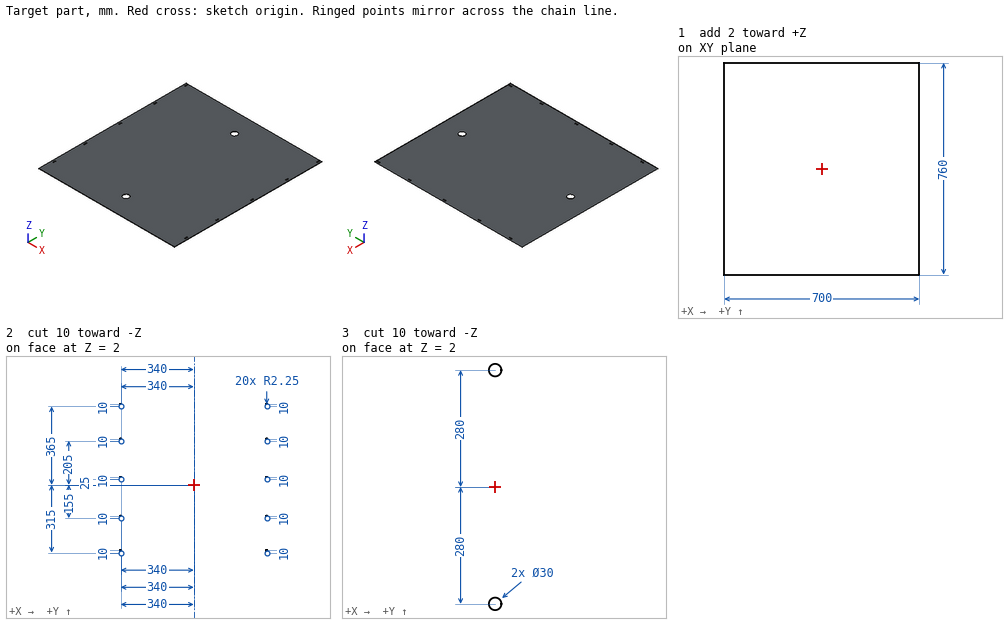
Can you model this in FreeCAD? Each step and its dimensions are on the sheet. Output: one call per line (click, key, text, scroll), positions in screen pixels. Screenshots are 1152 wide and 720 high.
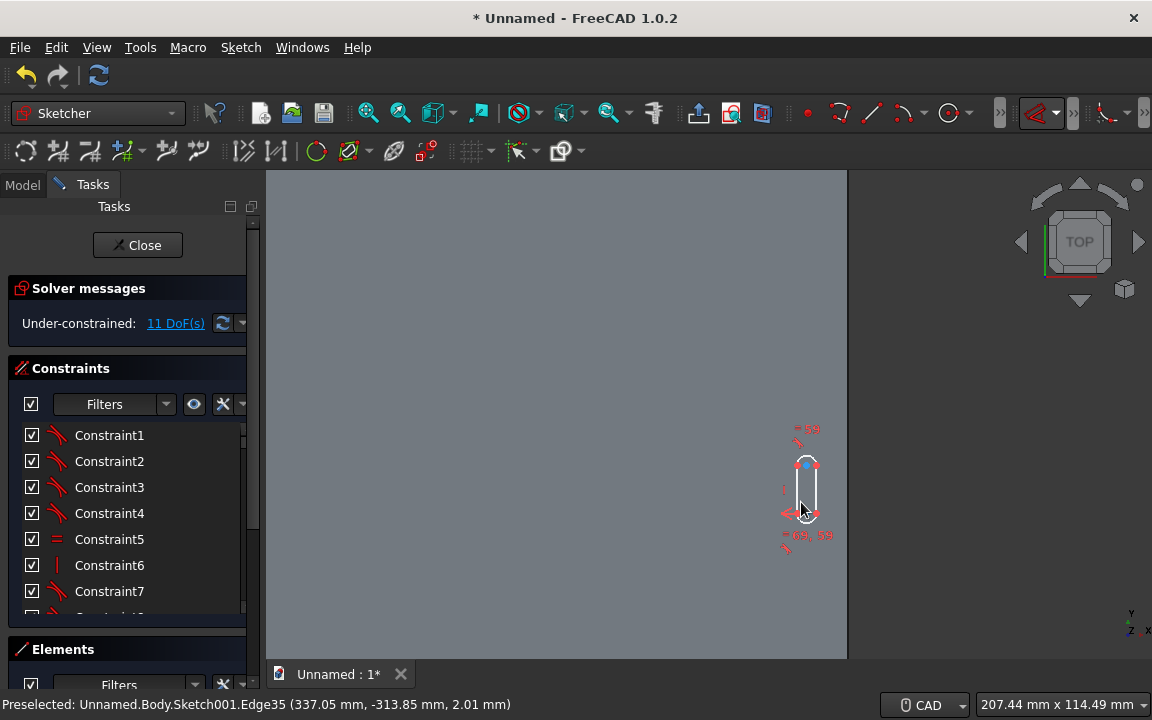
click(797, 499)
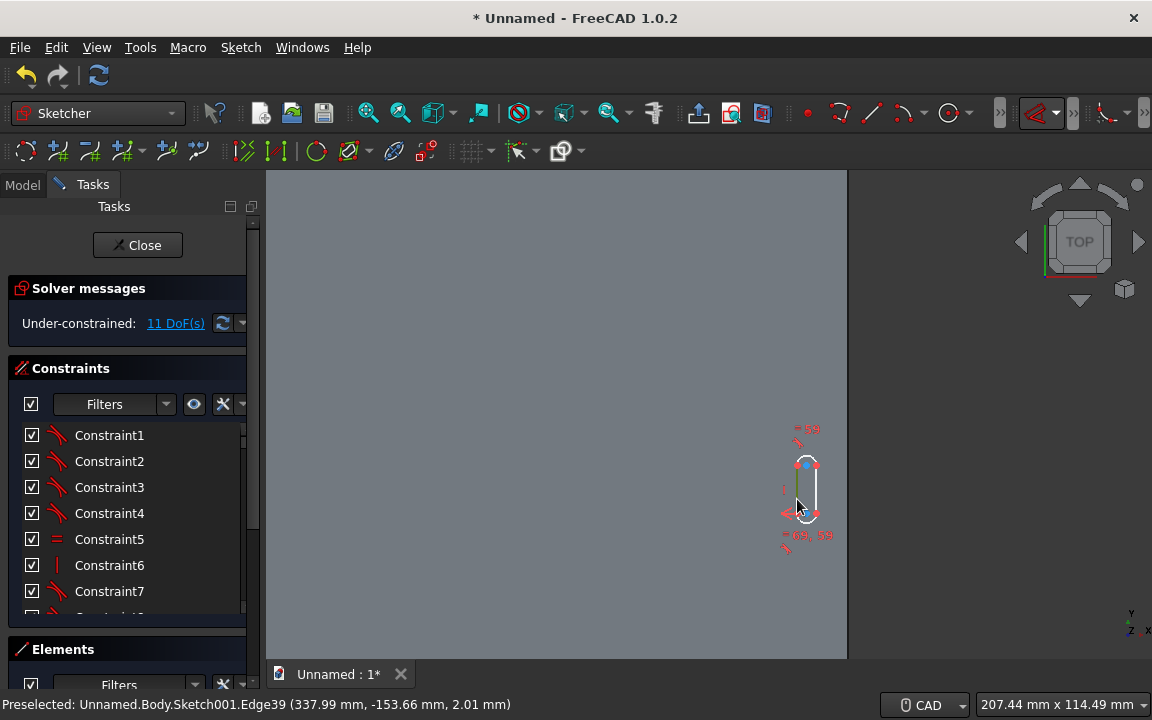
click(1058, 114)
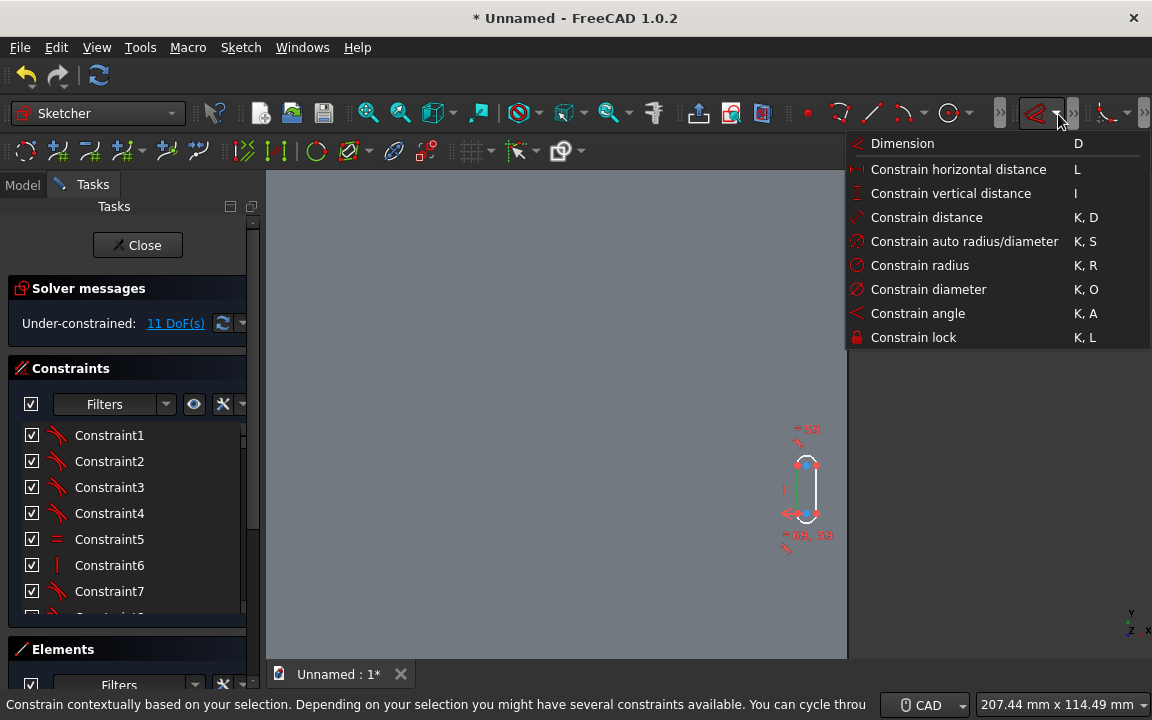
click(998, 193)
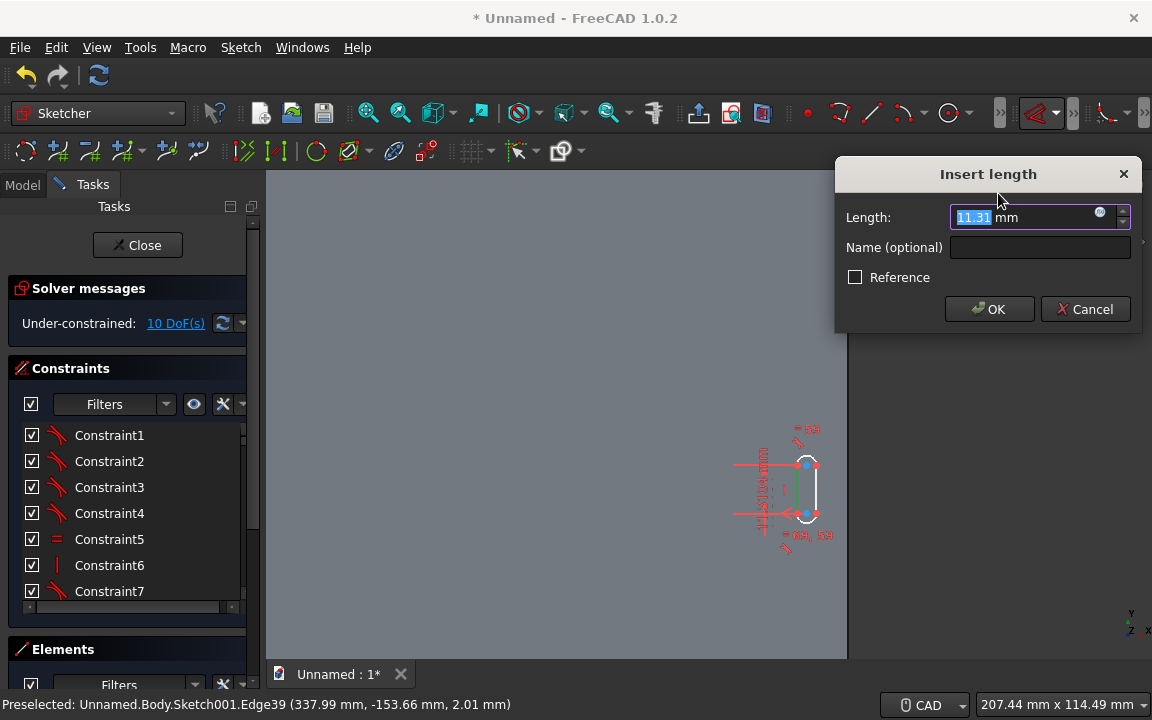
text(10)
key(Return)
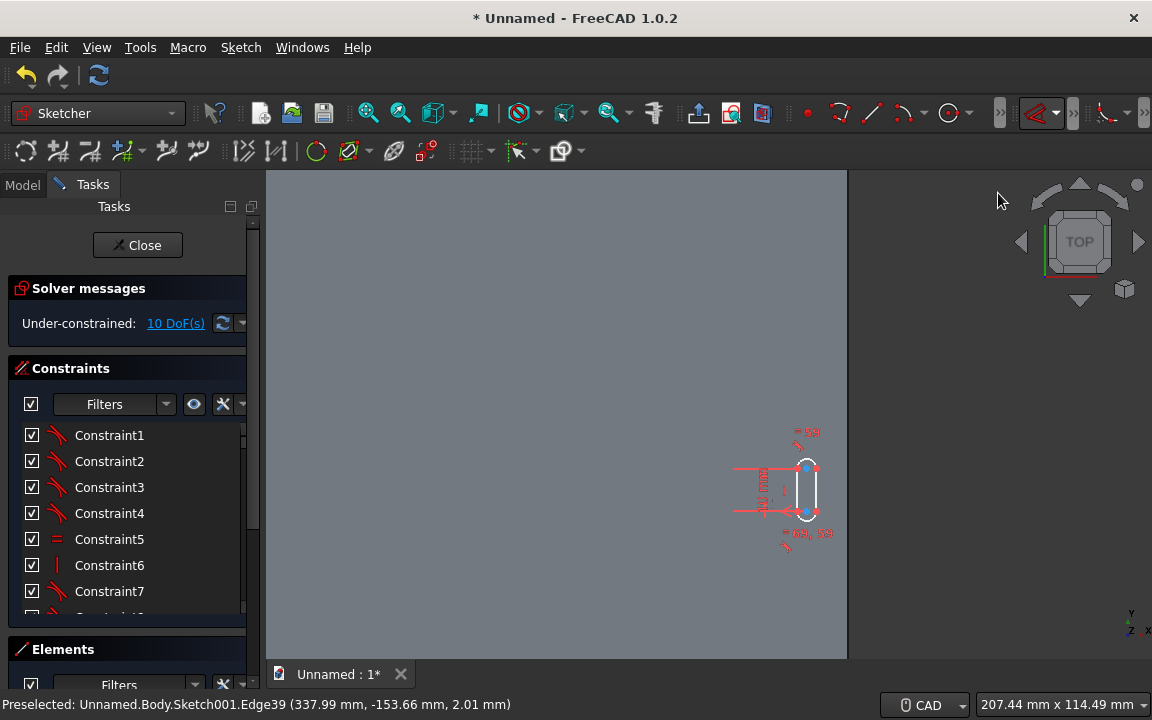
scroll(801, 502, down, 11)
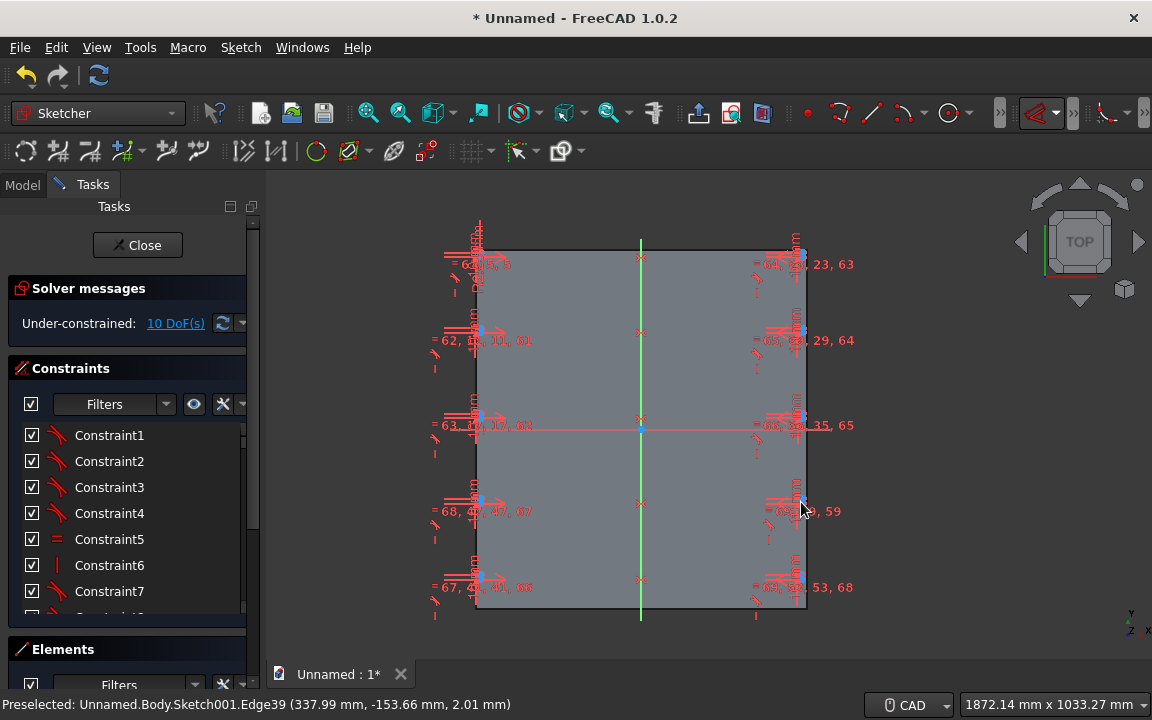
scroll(479, 418, up, 13)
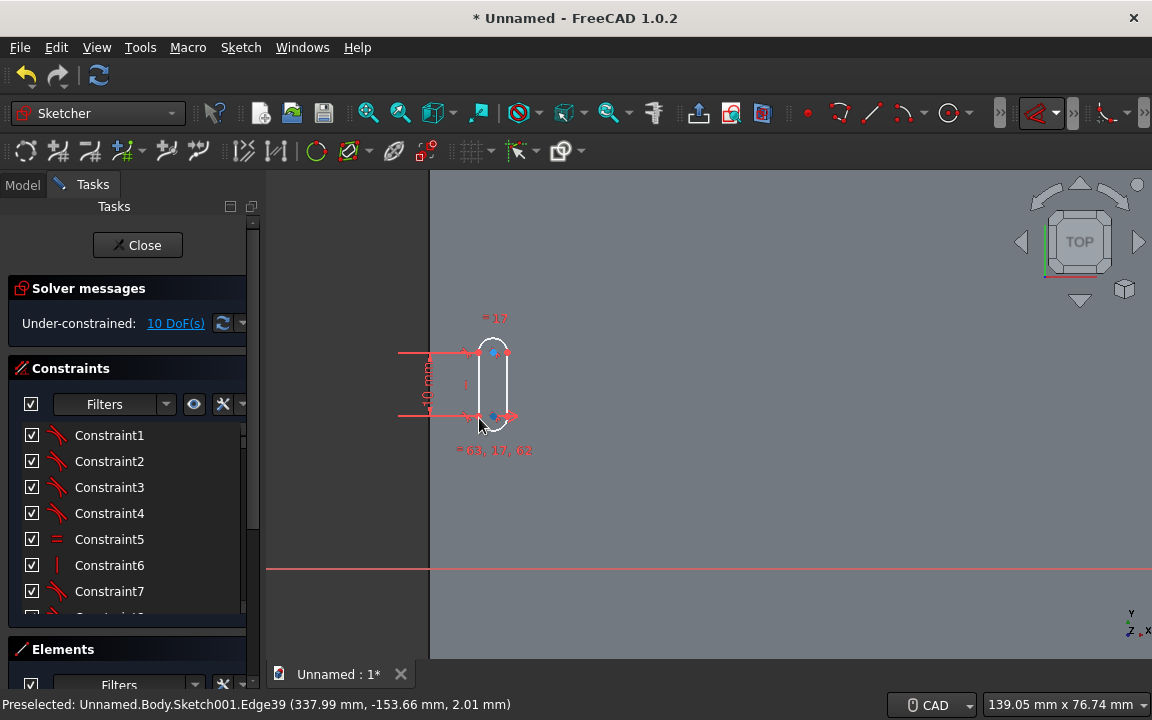
click(479, 416)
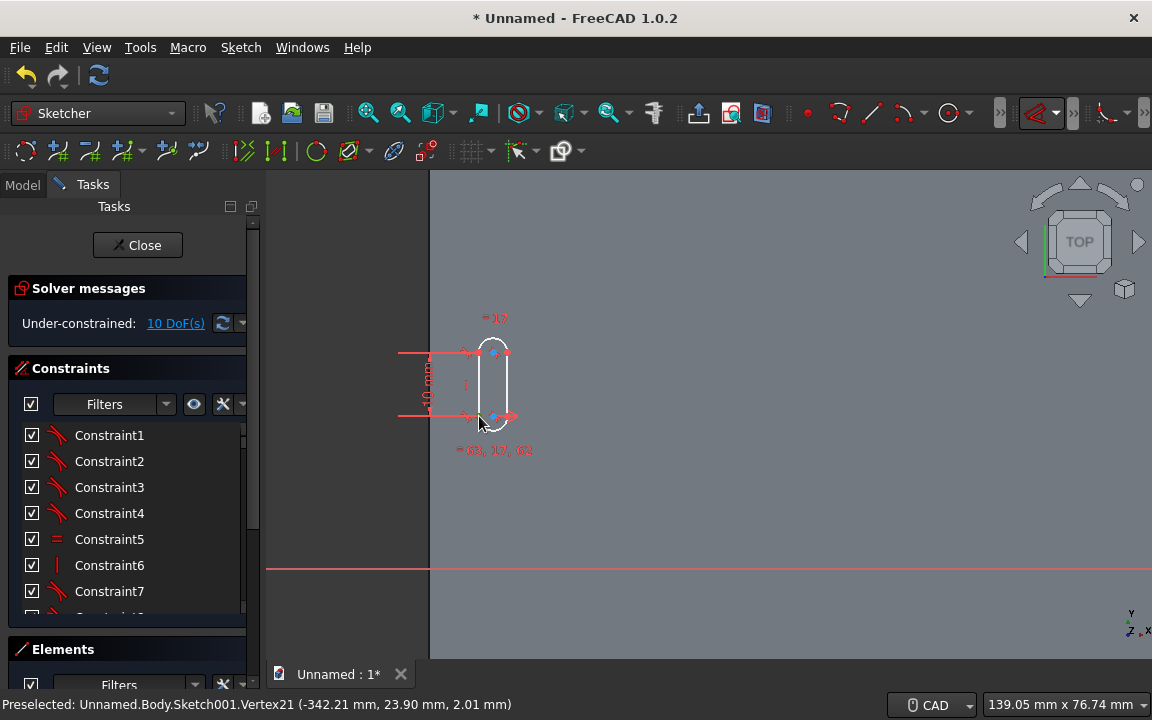
key(i)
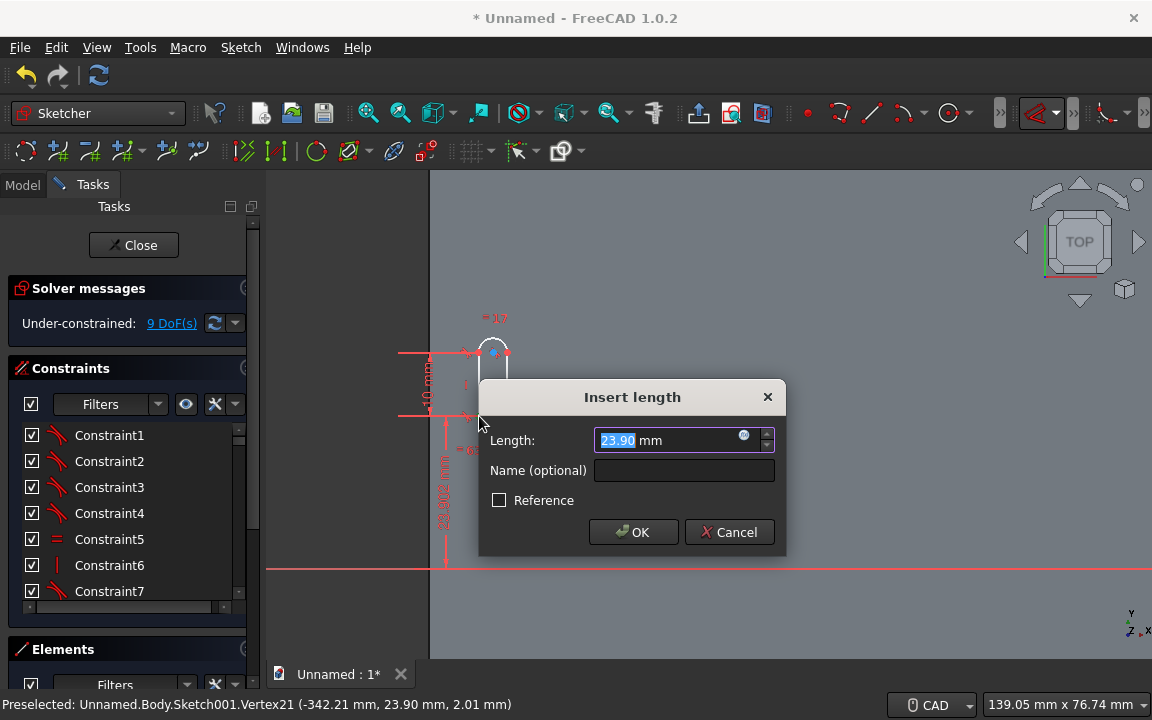
text(25)
key(Return)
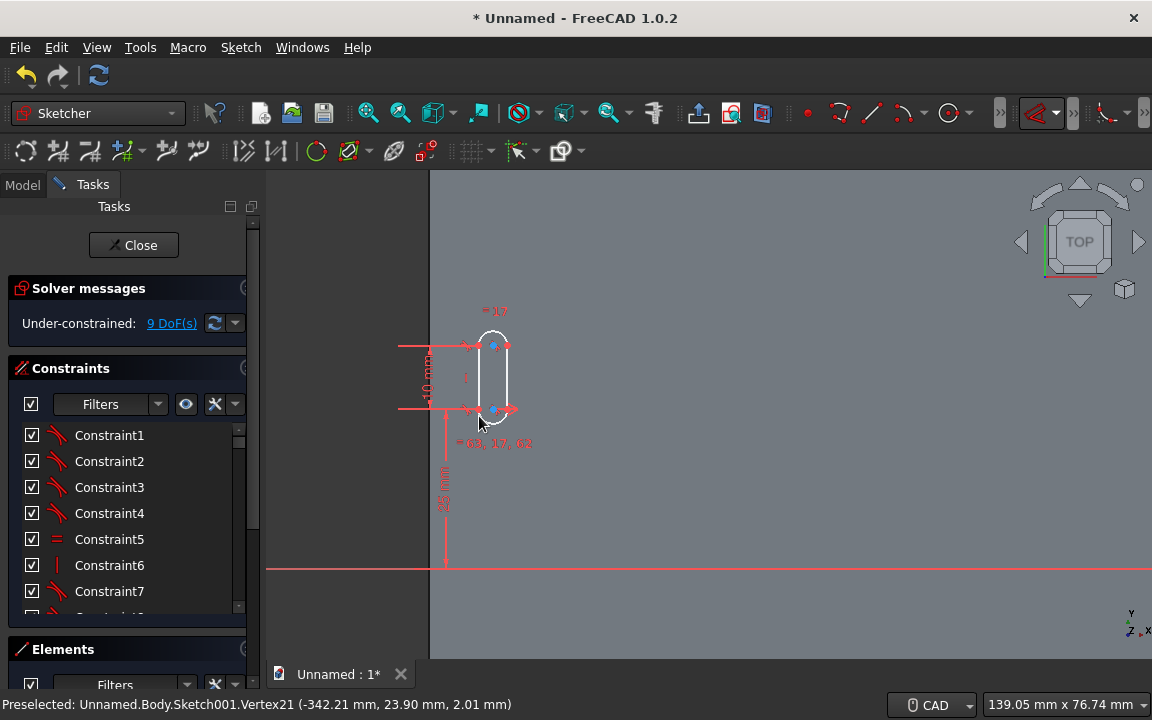
scroll(479, 417, down, 13)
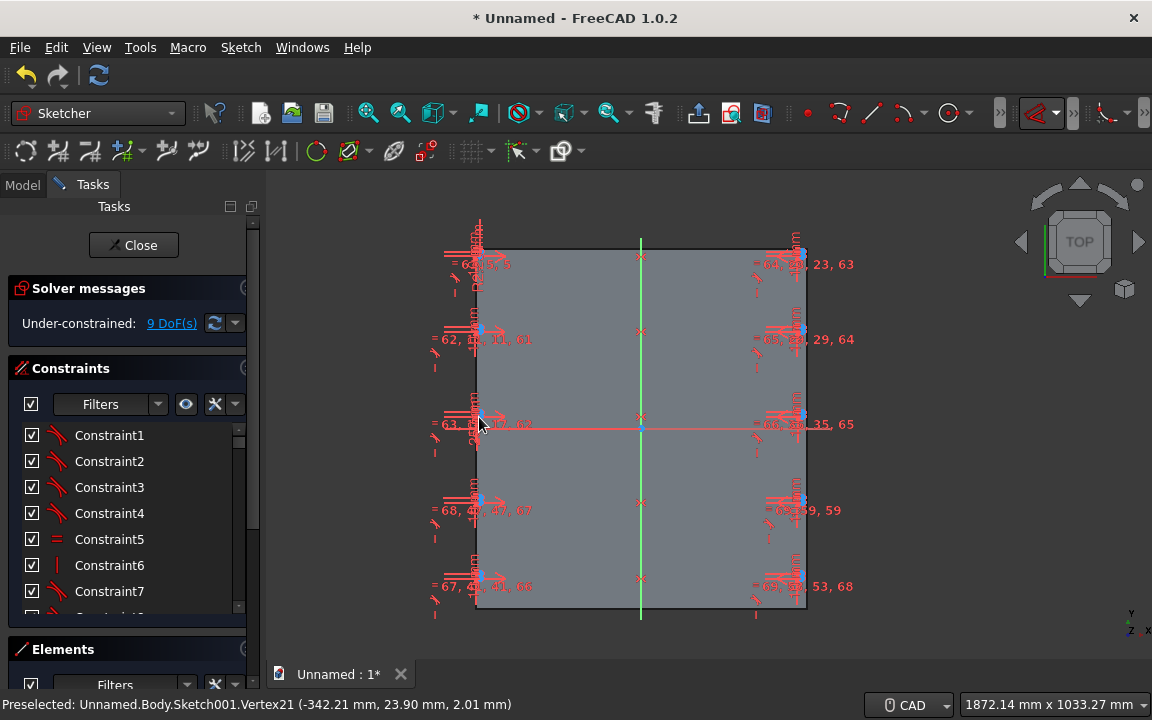
scroll(479, 256, up, 13)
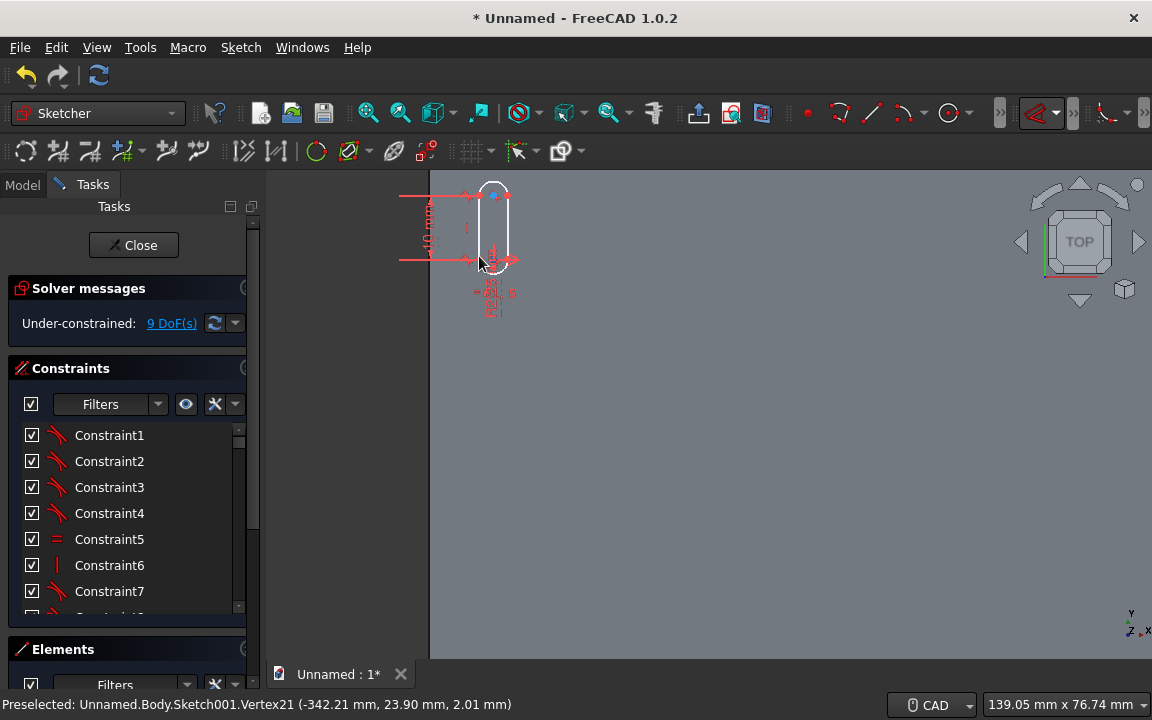
click(479, 260)